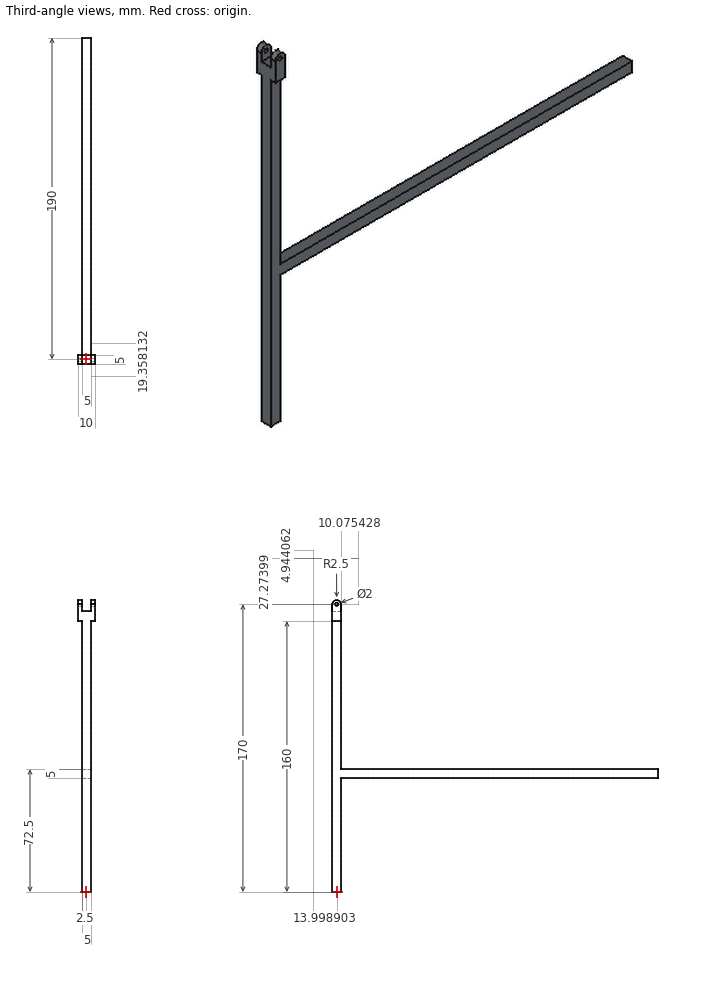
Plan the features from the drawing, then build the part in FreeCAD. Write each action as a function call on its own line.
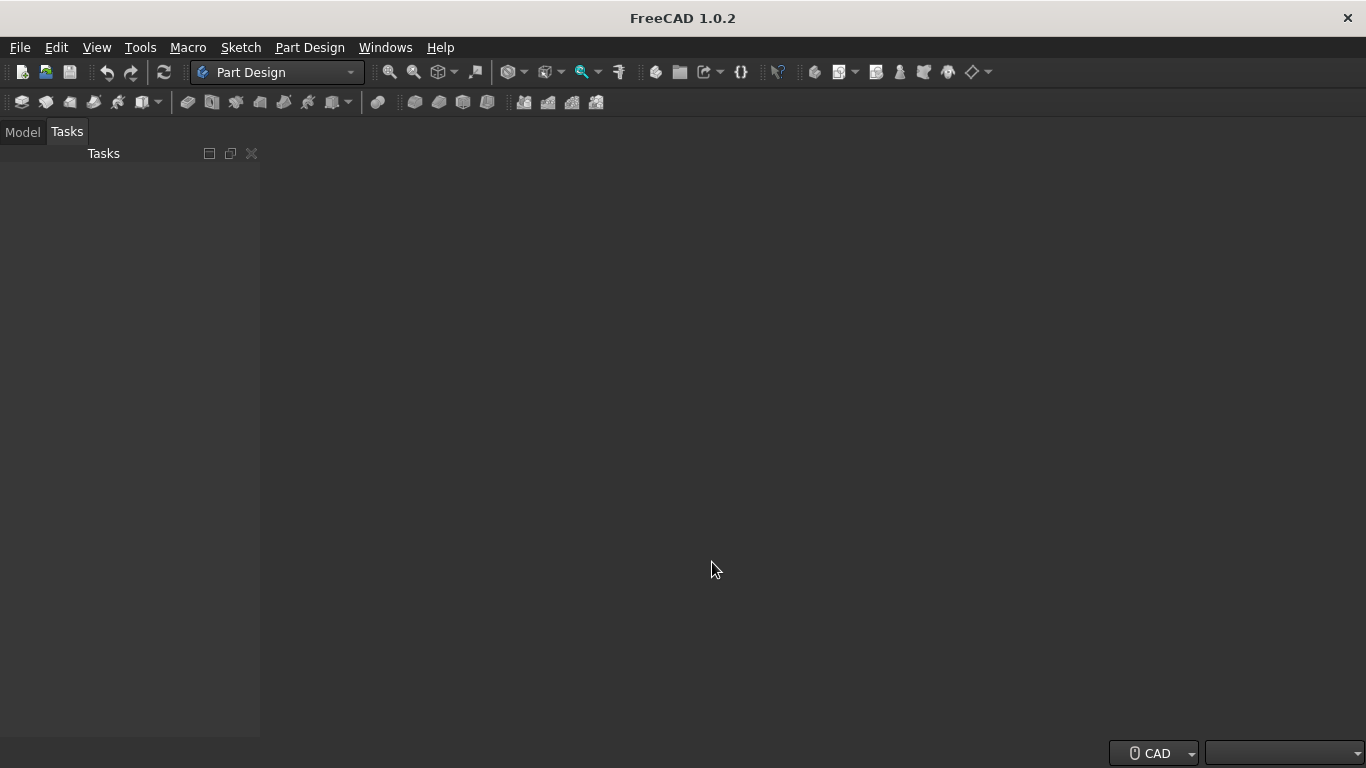
click(22, 72)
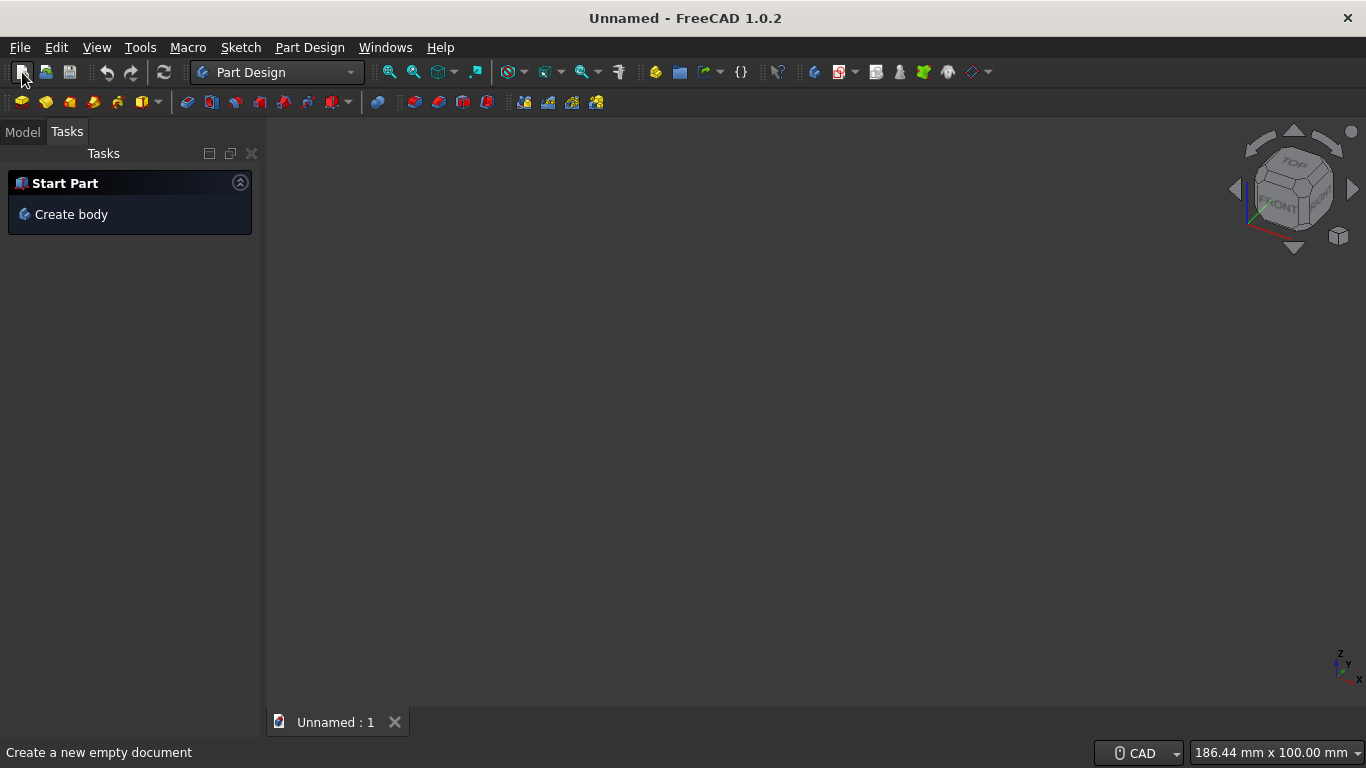
click(840, 72)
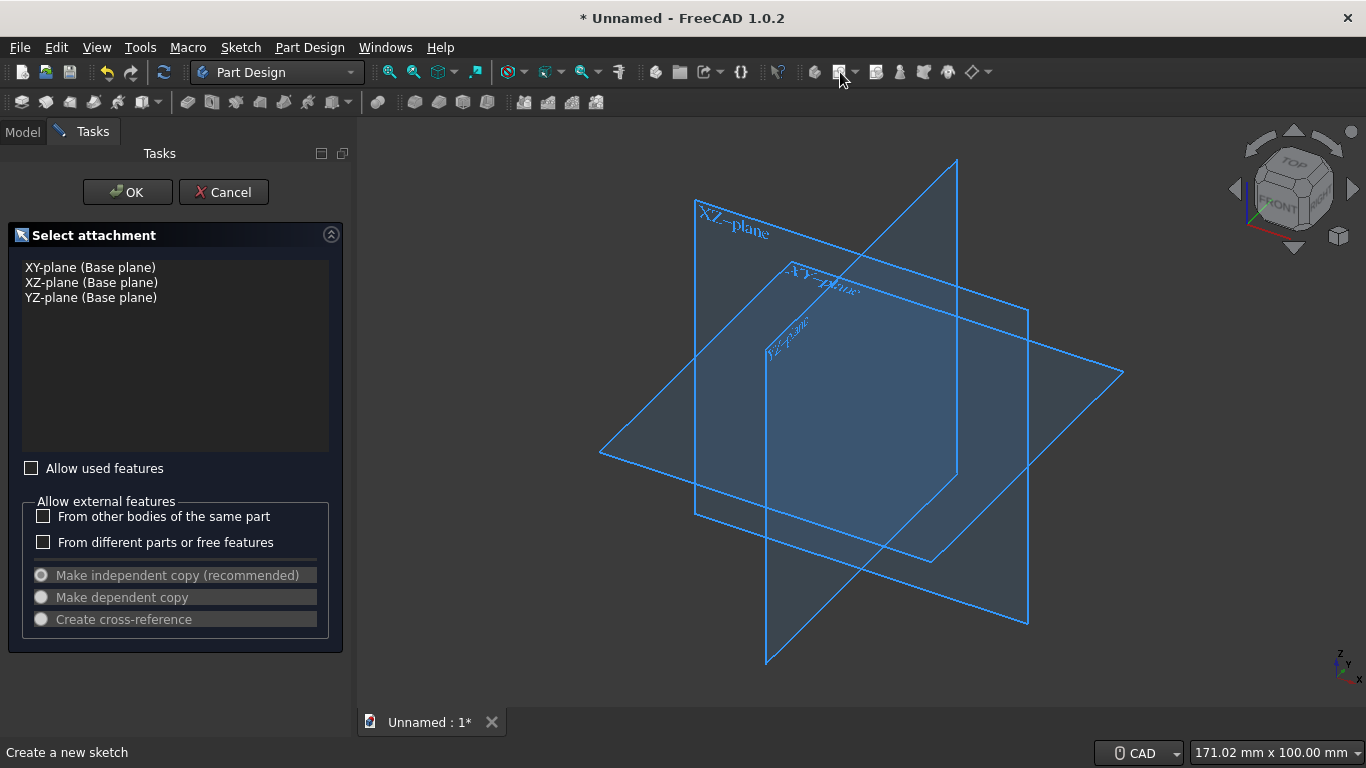
click(82, 268)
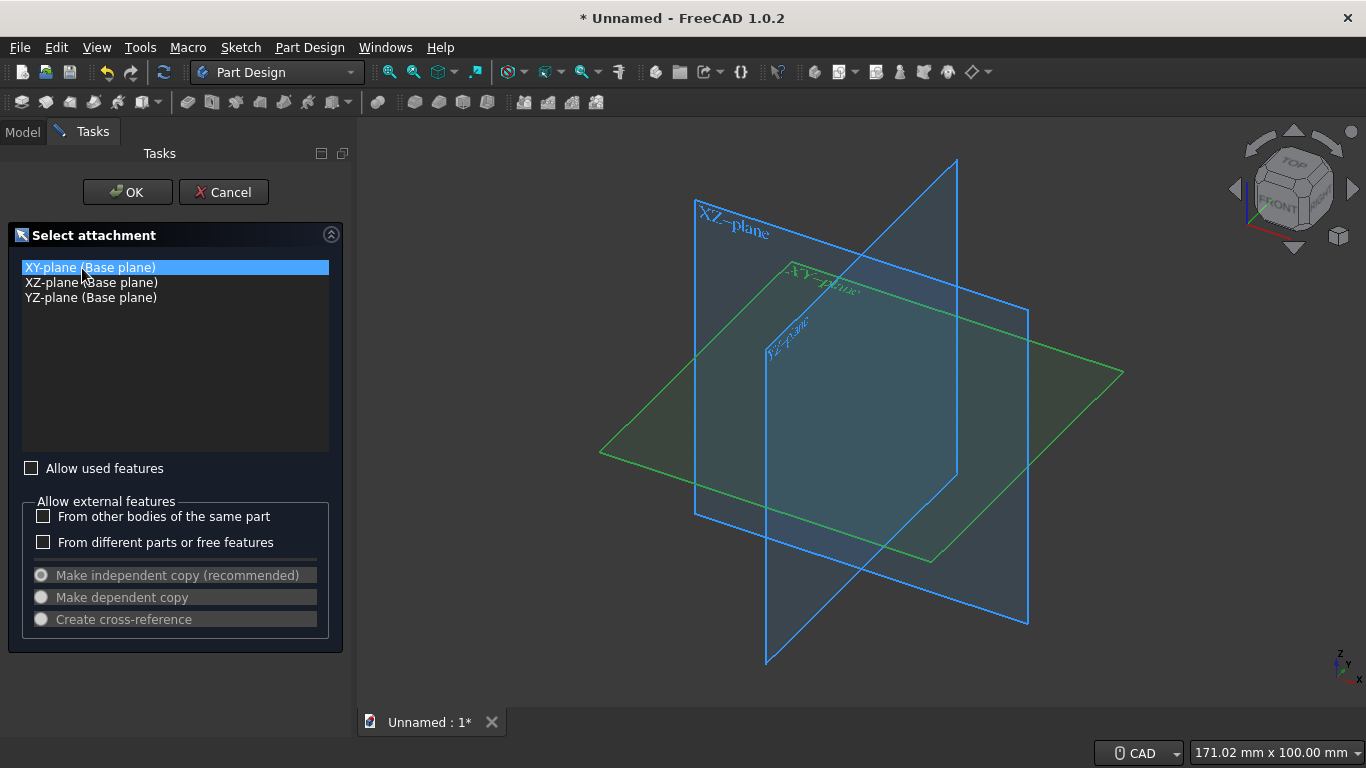
click(128, 192)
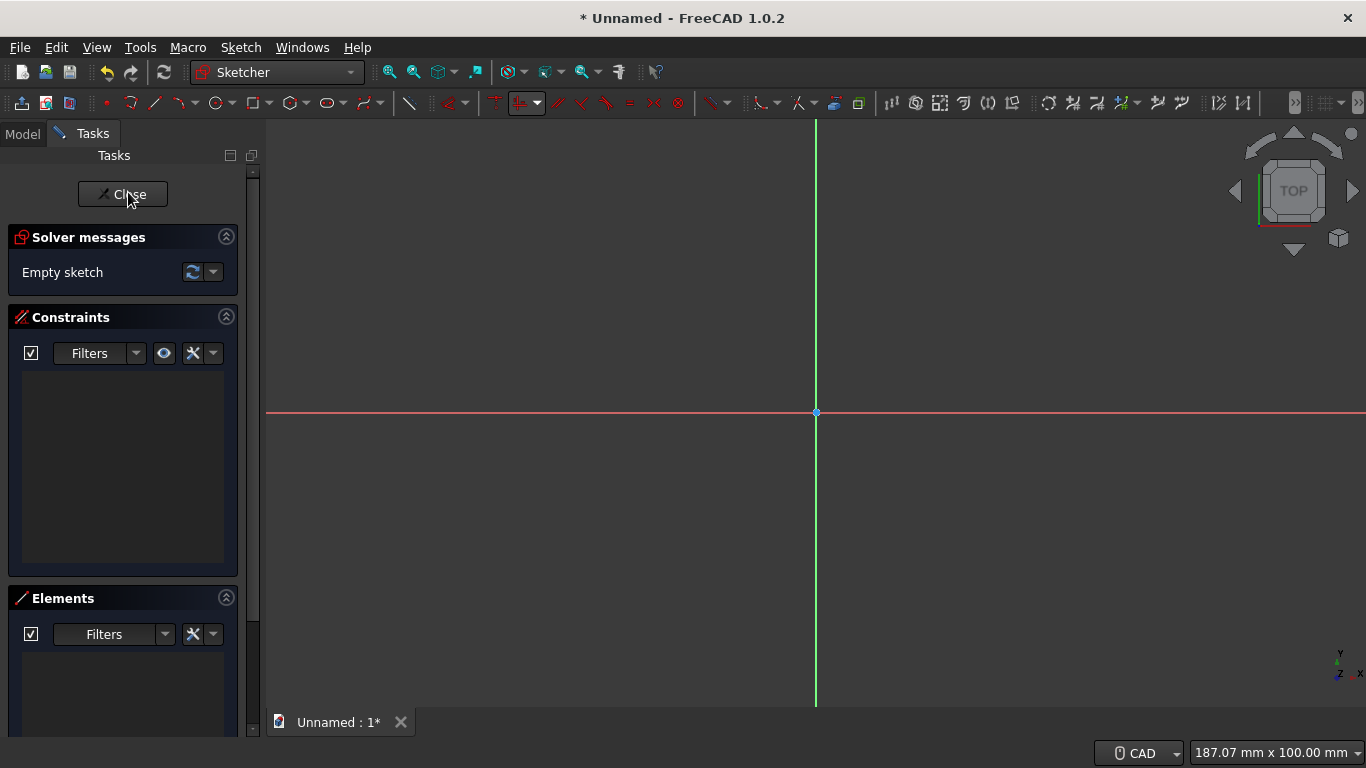
scroll(821, 413, up, 13)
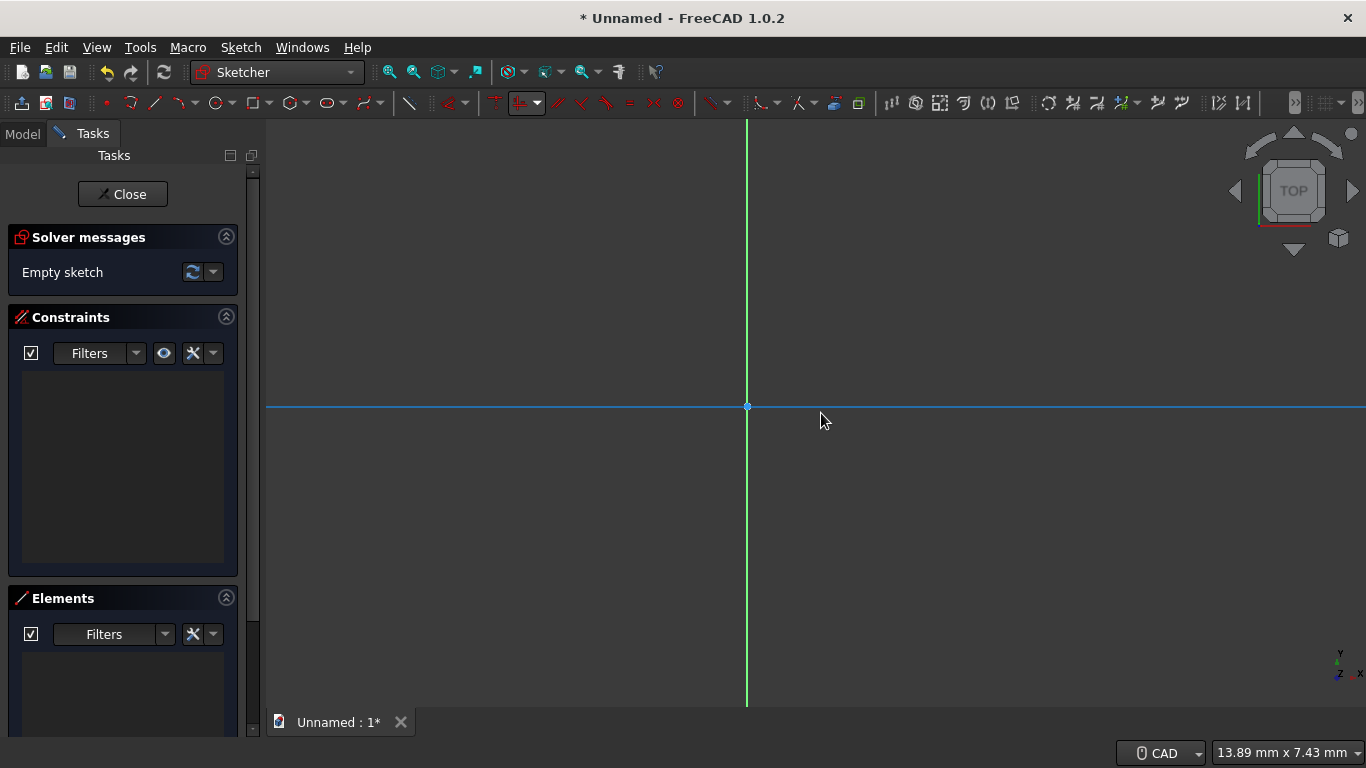
click(272, 104)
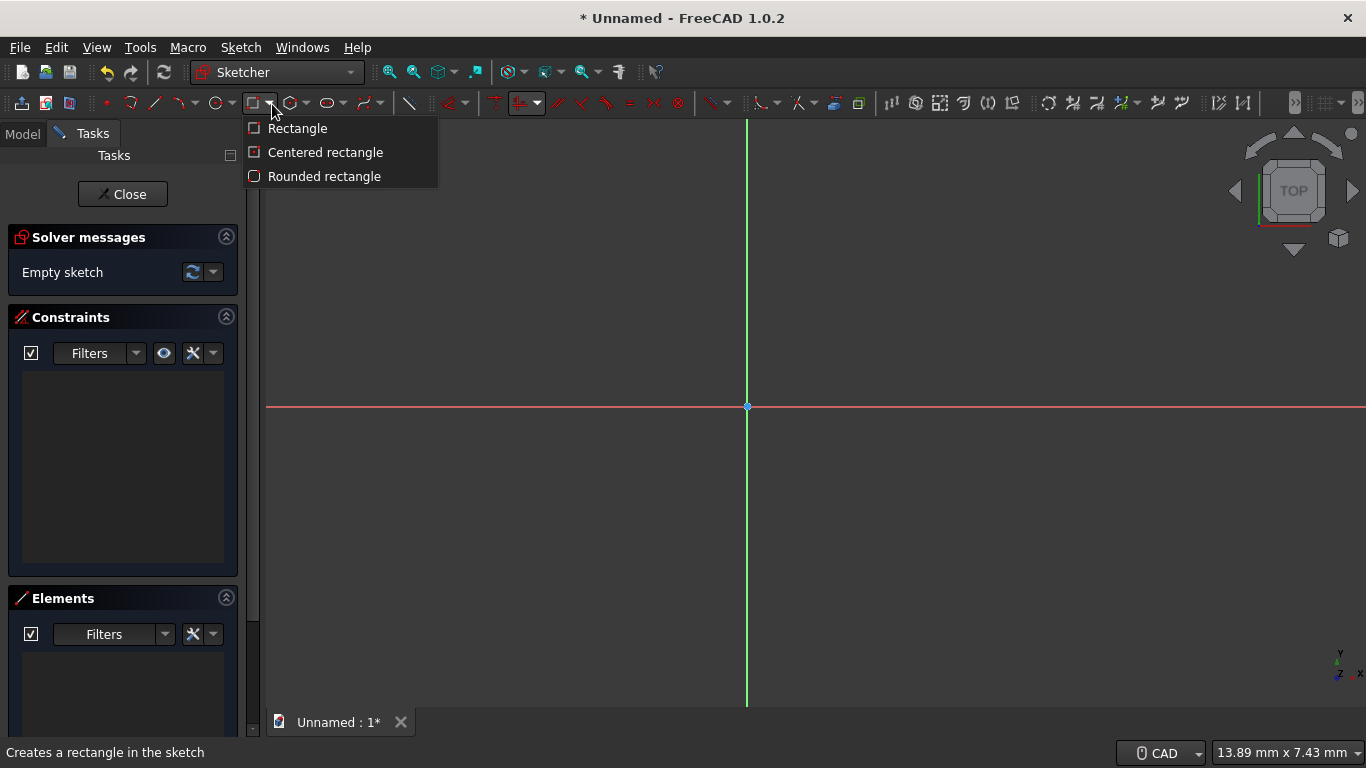
click(340, 152)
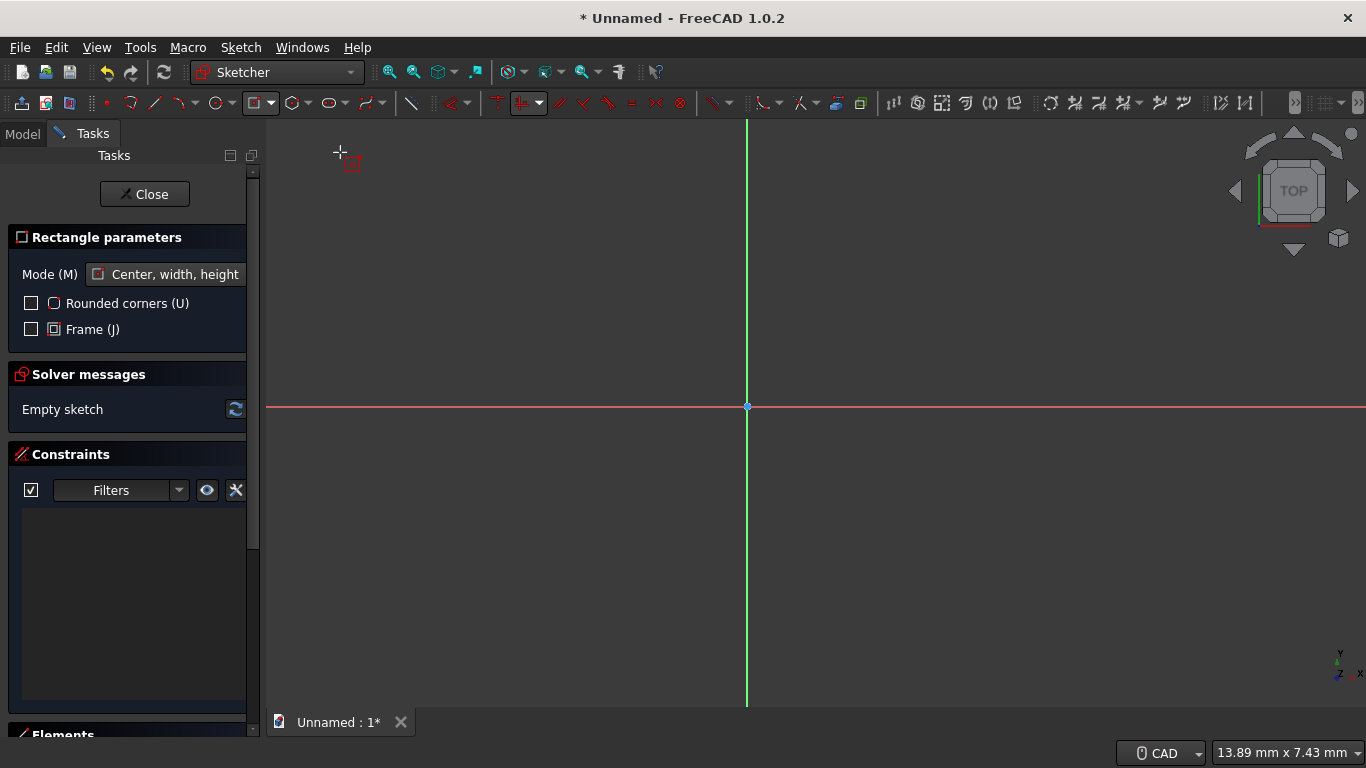
click(747, 407)
click(945, 209)
key(Escape)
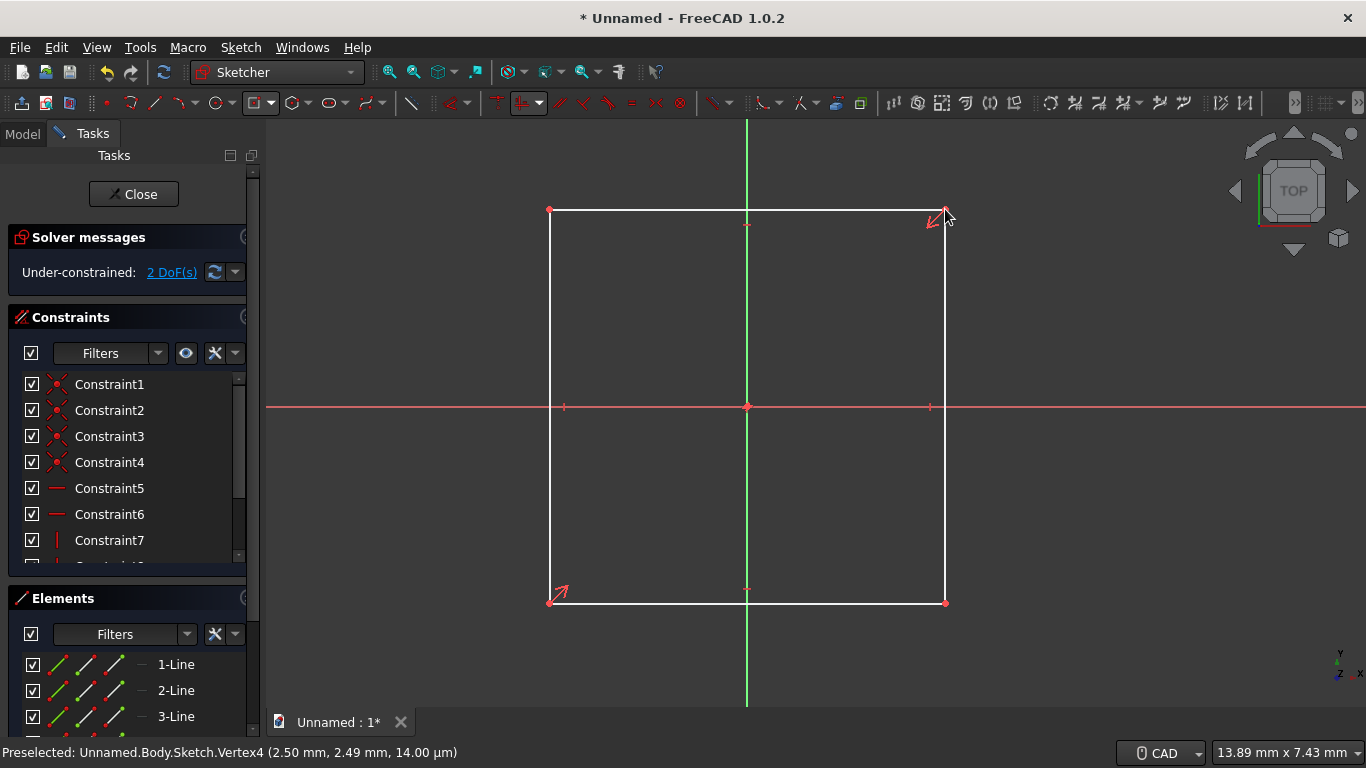
click(668, 604)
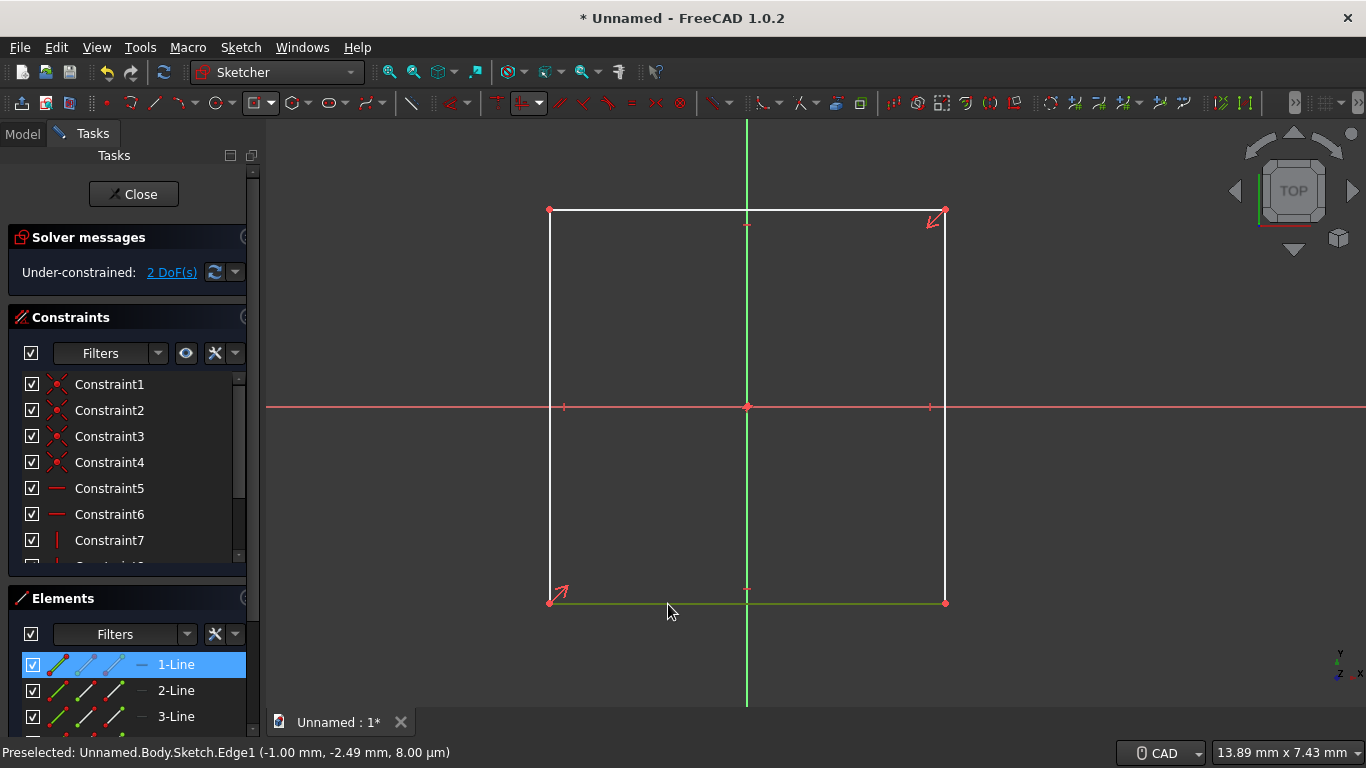
click(470, 104)